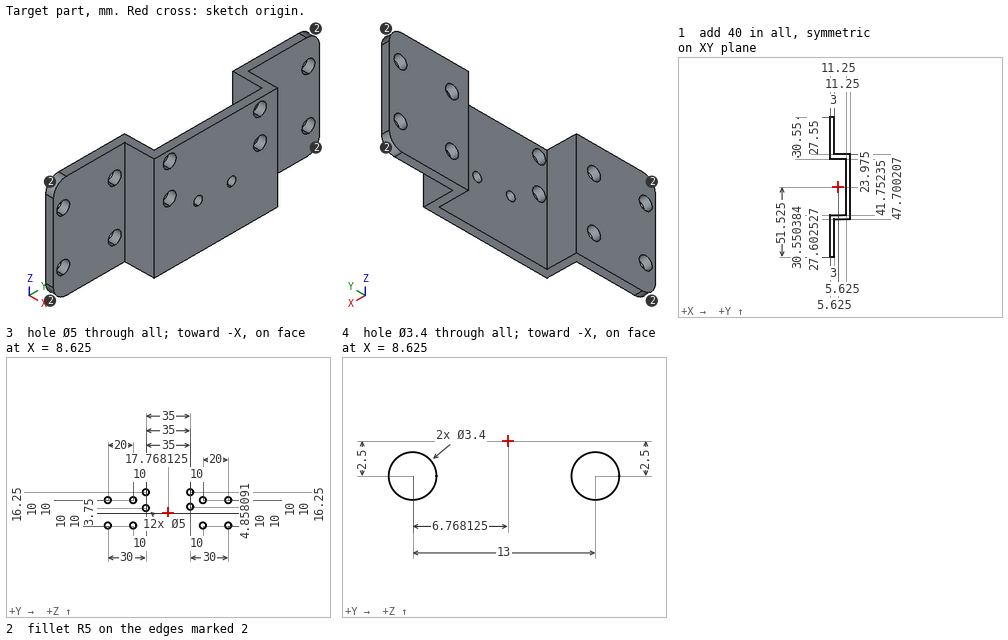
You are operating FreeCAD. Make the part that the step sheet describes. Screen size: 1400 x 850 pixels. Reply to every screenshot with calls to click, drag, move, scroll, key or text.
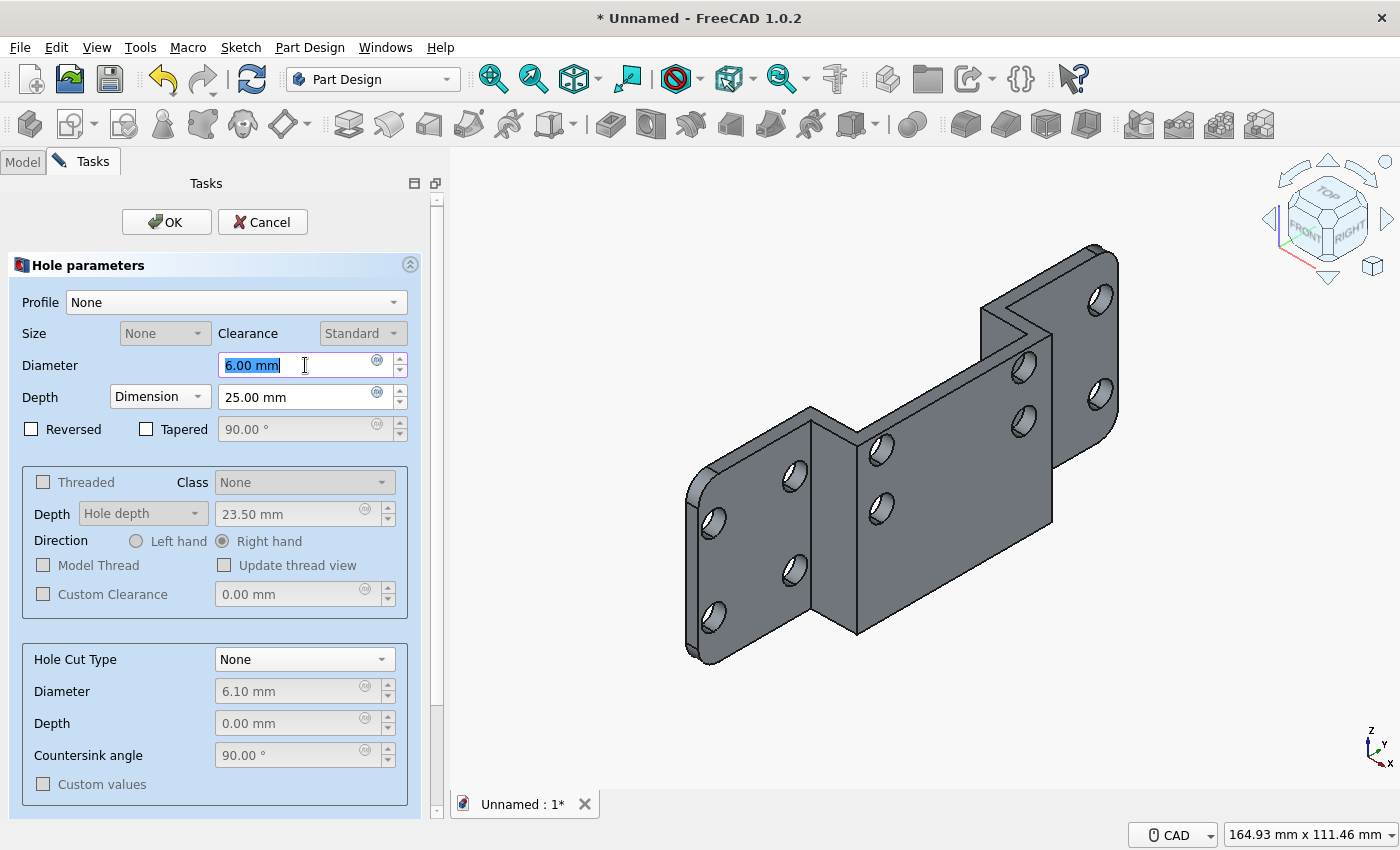
text(5)
key(Tab)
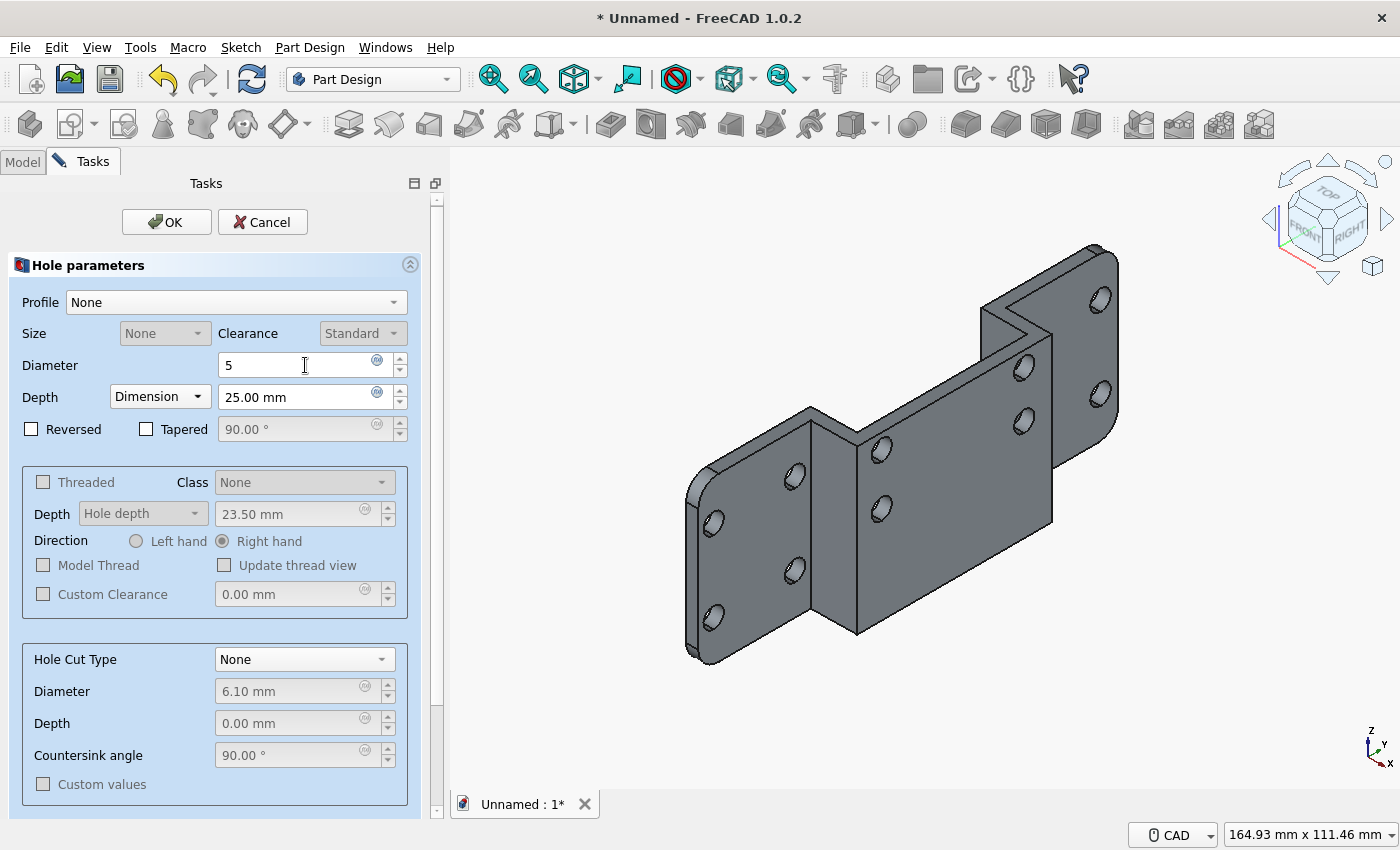
click(161, 396)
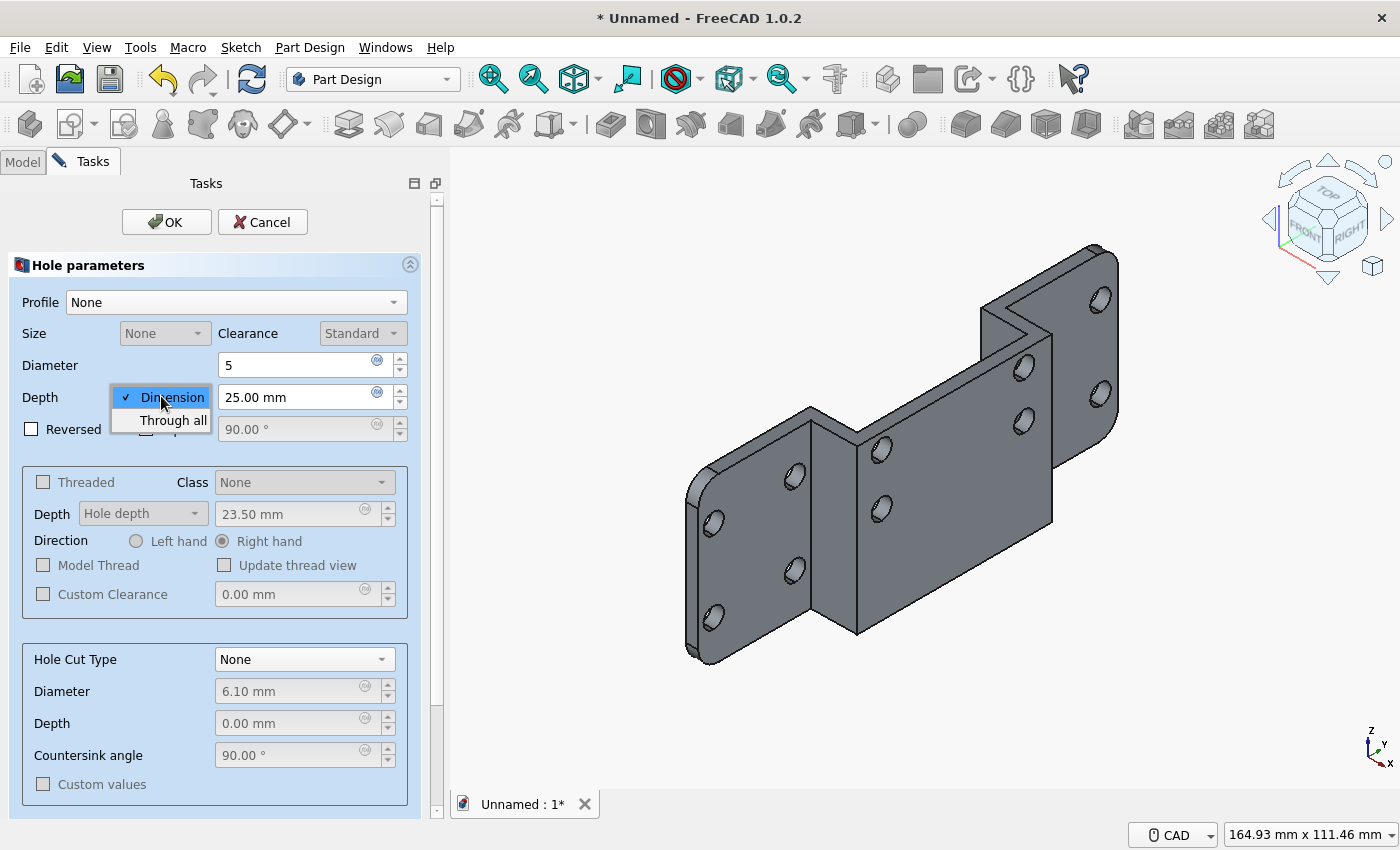
click(160, 420)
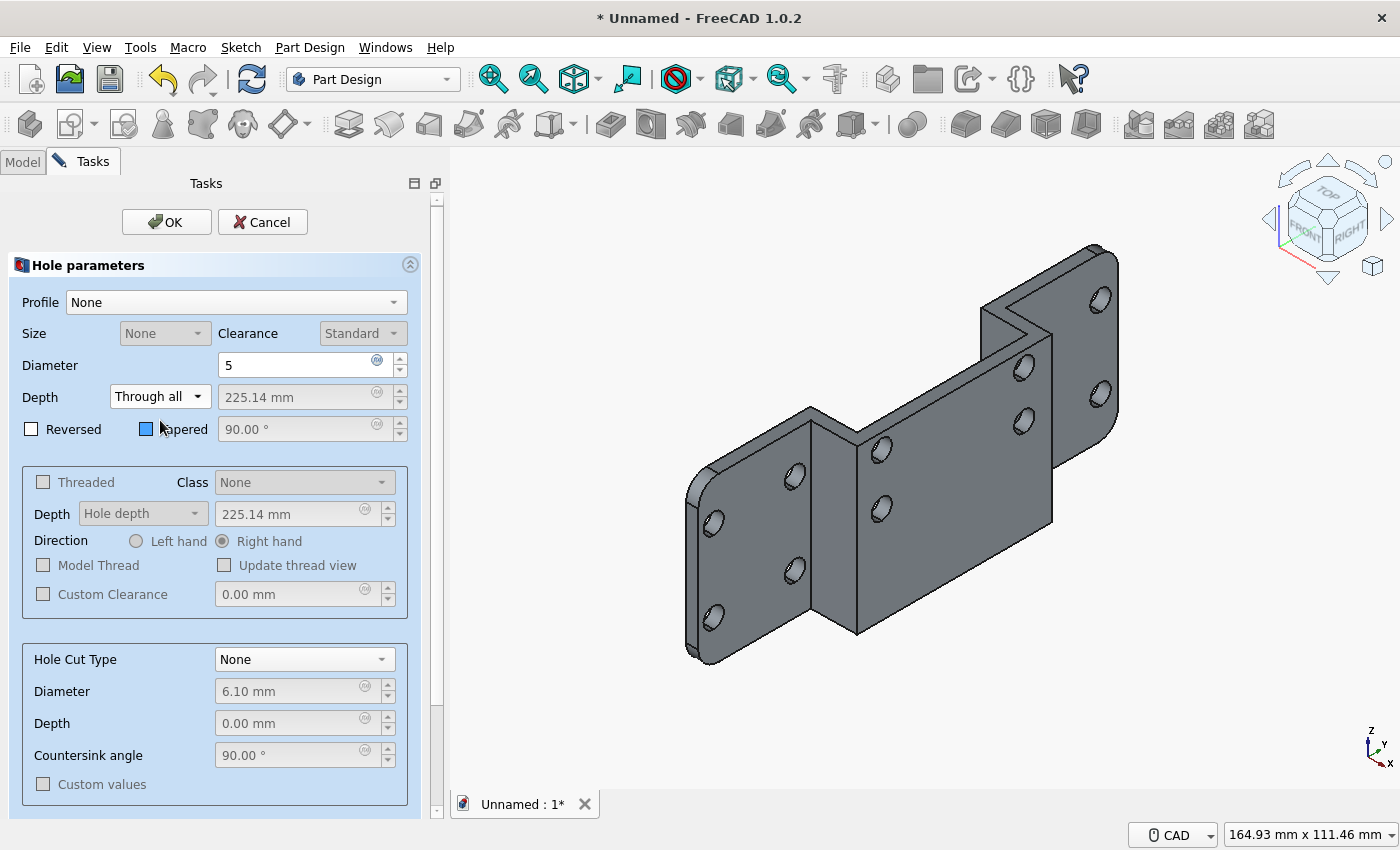
click(167, 222)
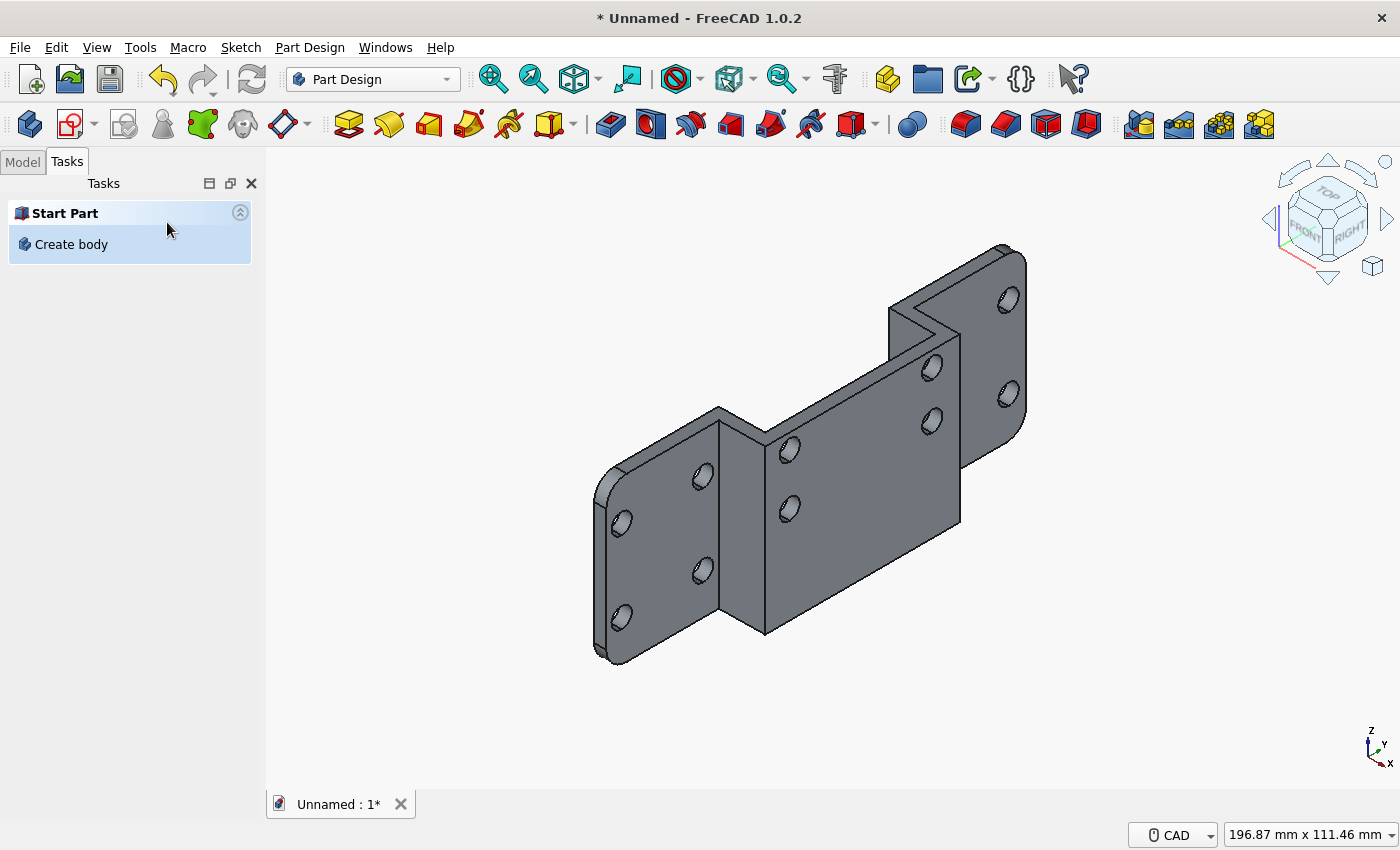
click(863, 483)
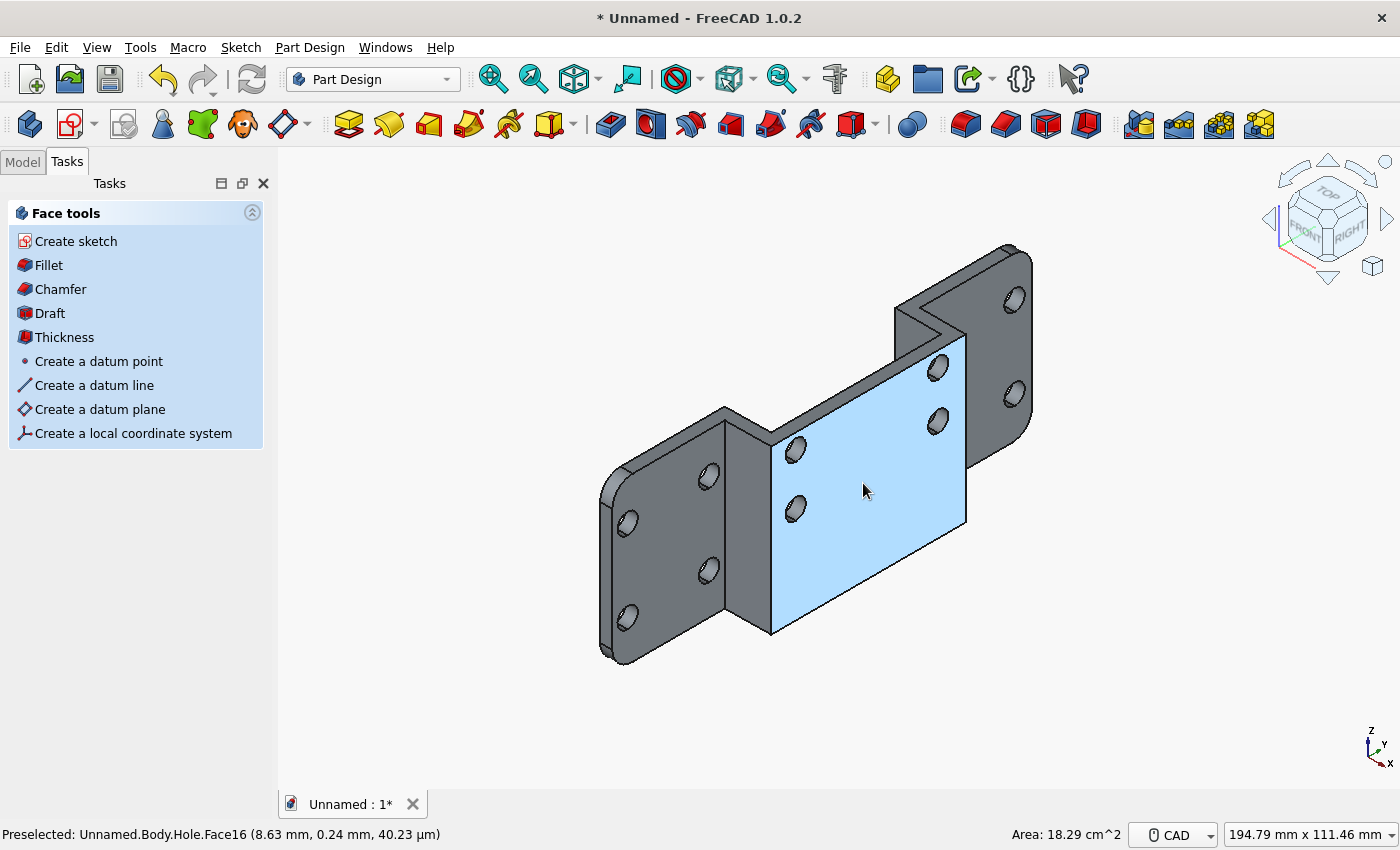
click(70, 124)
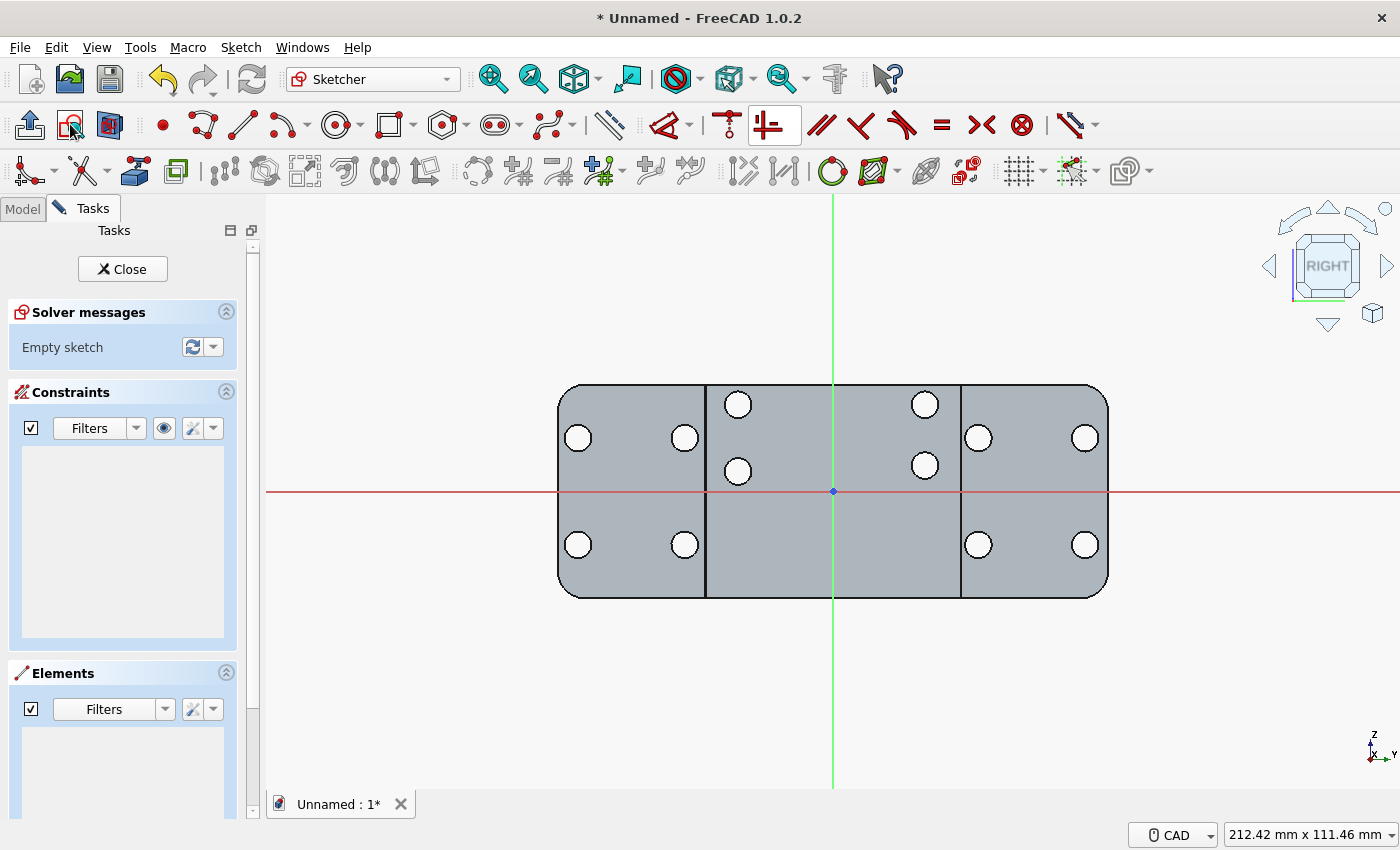
scroll(842, 504, up, 10)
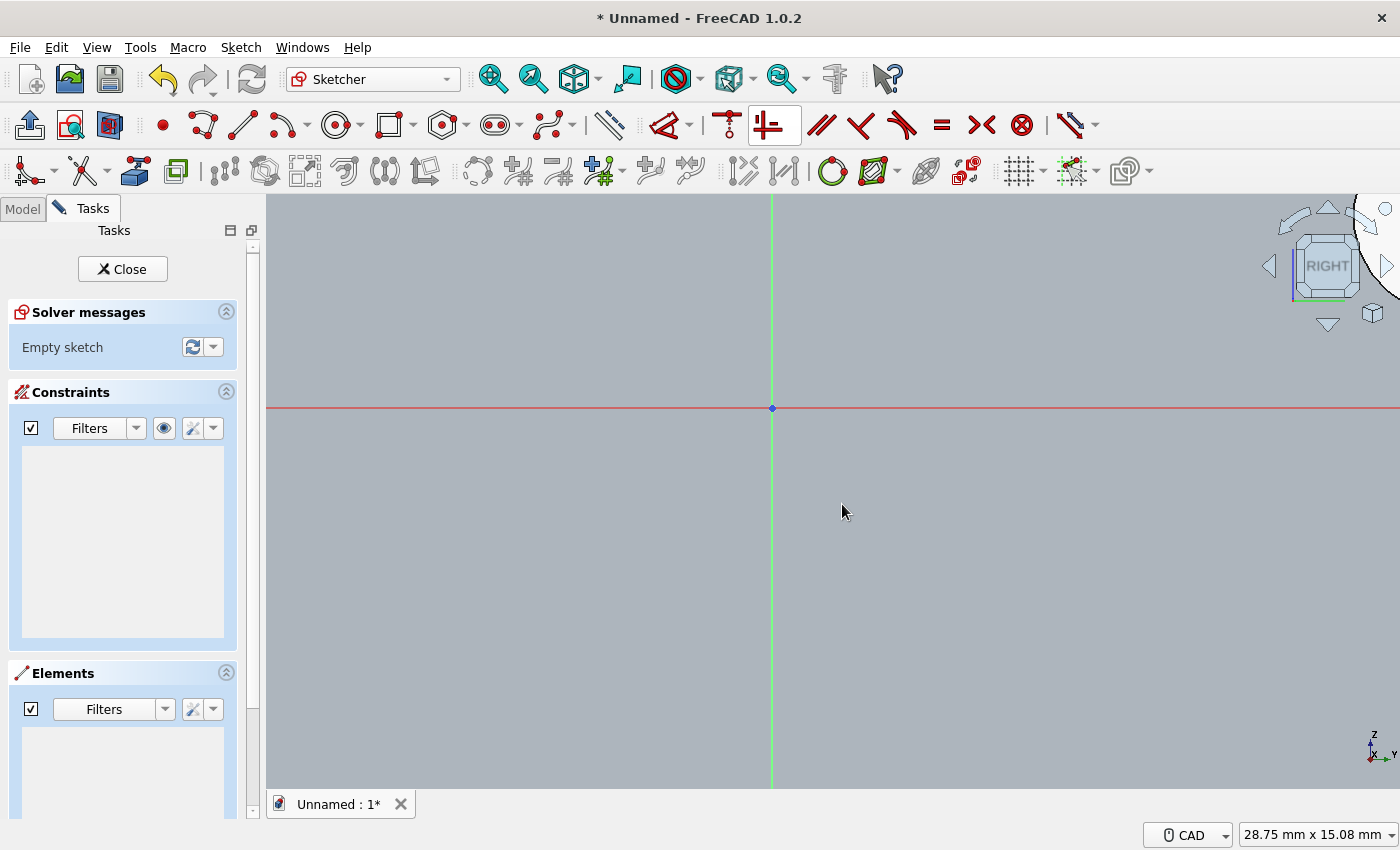
click(336, 126)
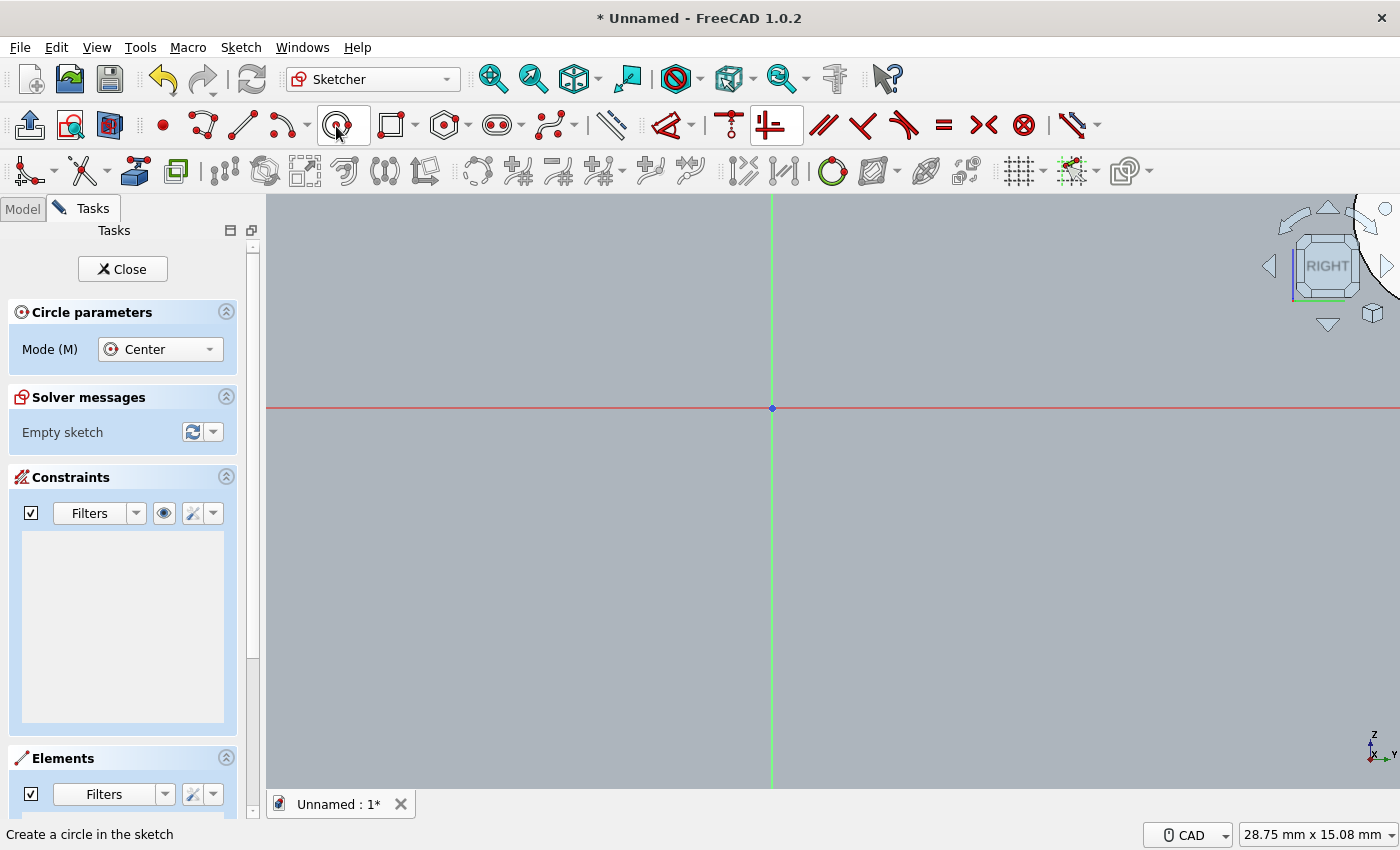
click(505, 507)
click(553, 460)